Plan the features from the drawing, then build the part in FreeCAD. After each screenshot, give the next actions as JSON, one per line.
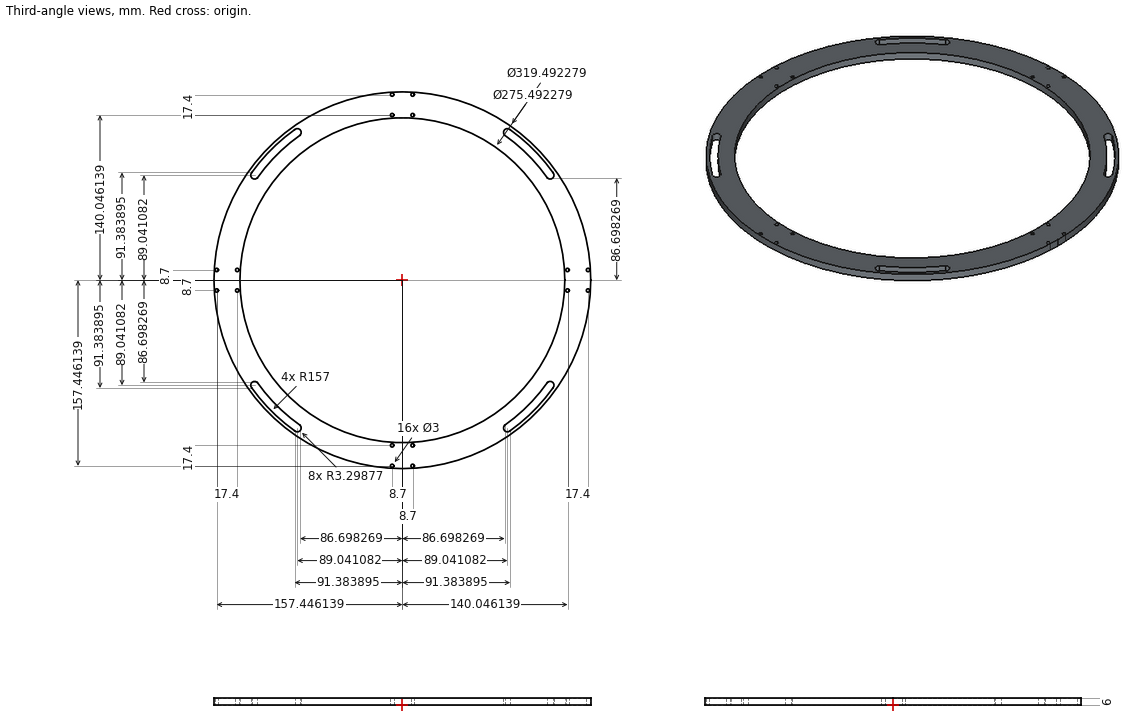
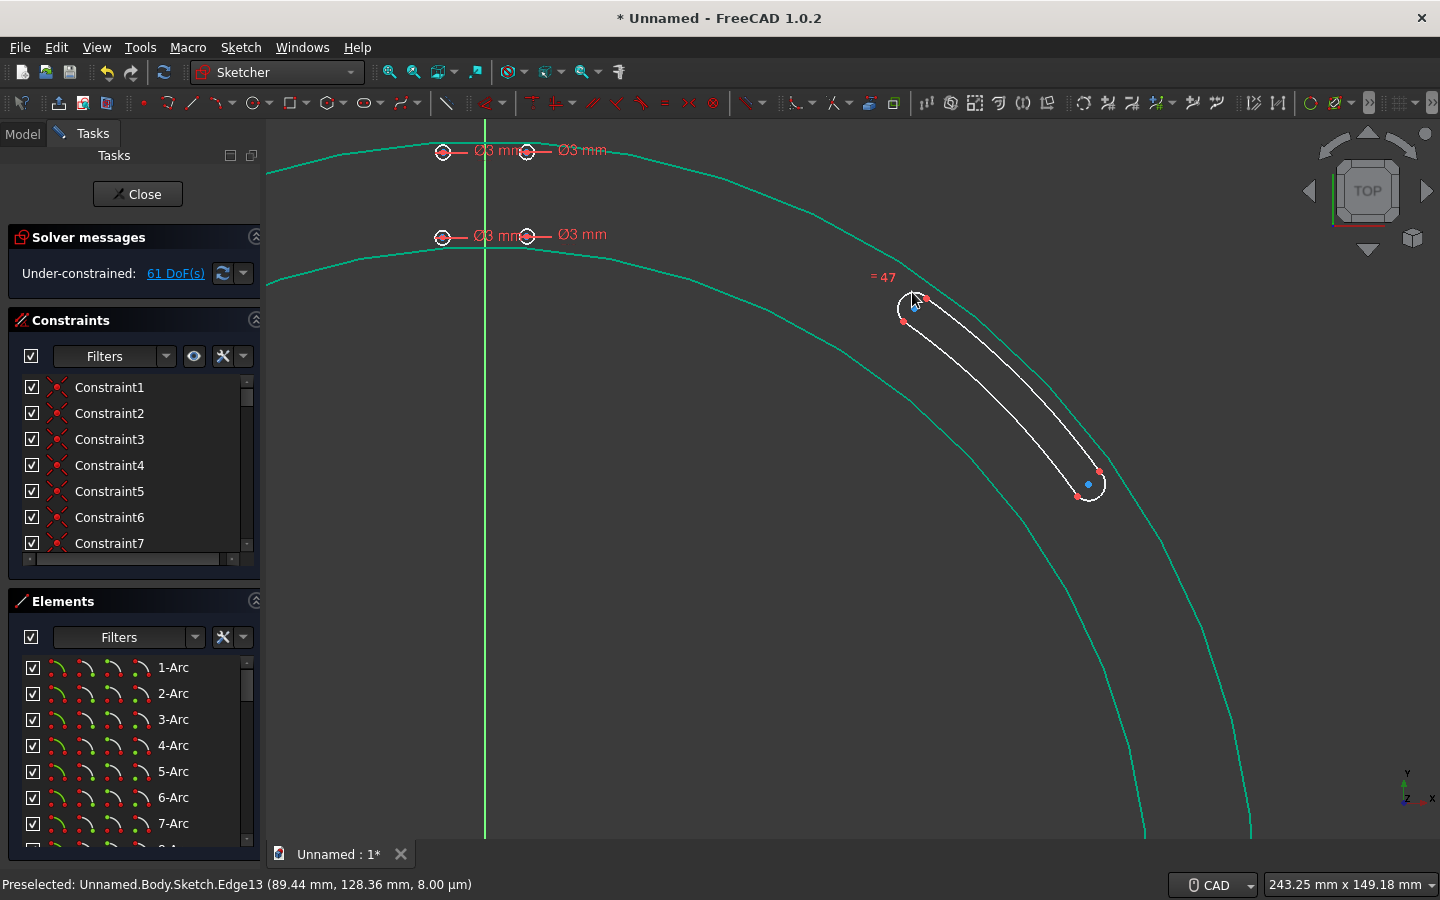
{"action": "scroll", "coordinate": [914, 292], "scroll_direction": "down", "scroll_amount": 6}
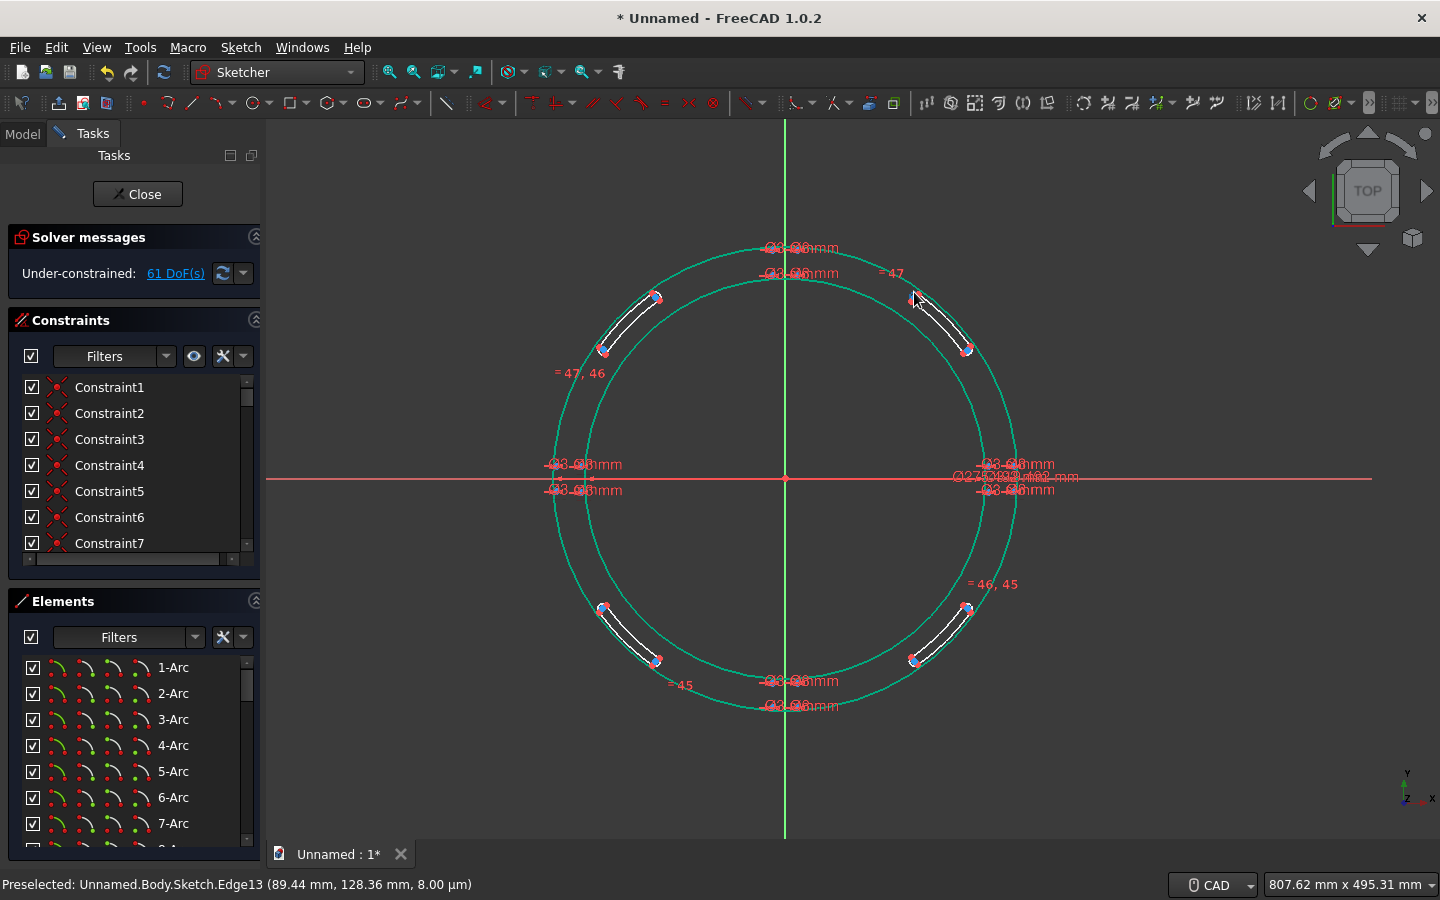
{"action": "scroll", "coordinate": [613, 630], "scroll_direction": "up", "scroll_amount": 7}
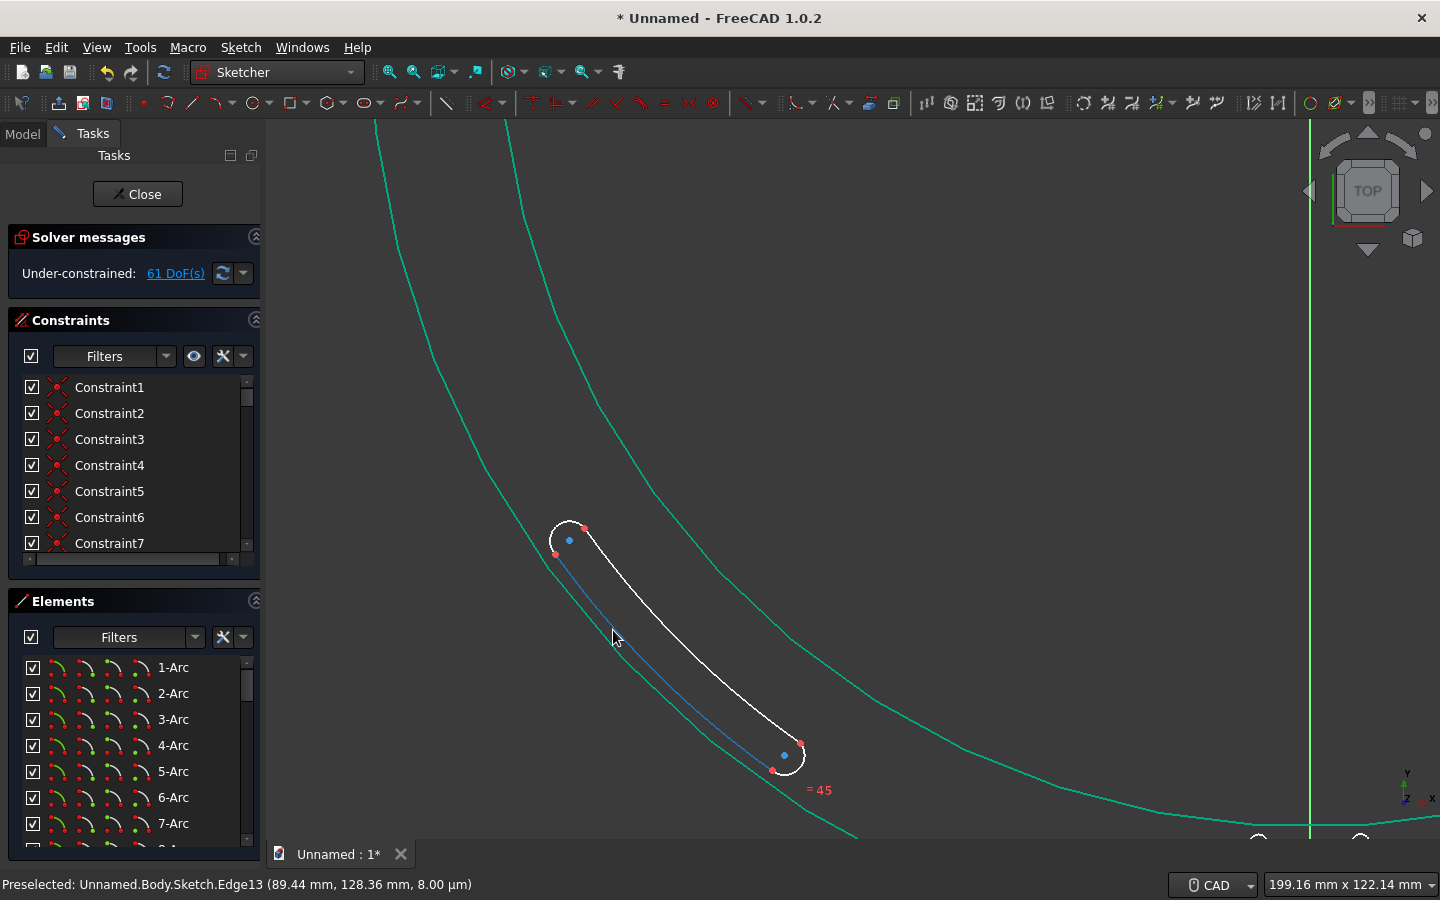
{"action": "left_click", "coordinate": [613, 627]}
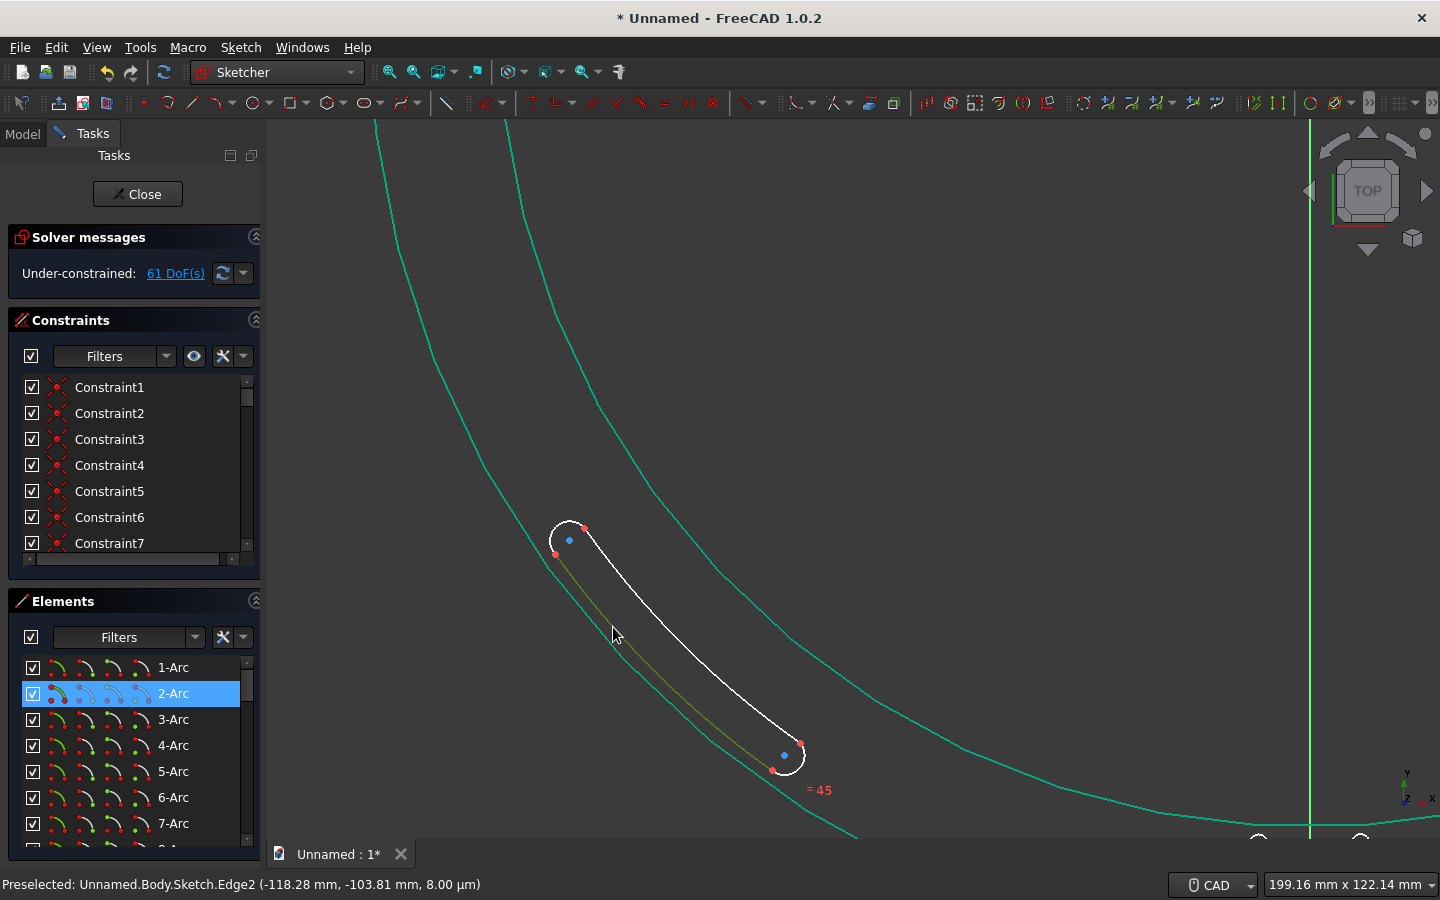
{"action": "scroll", "coordinate": [612, 631], "scroll_direction": "down", "scroll_amount": 7}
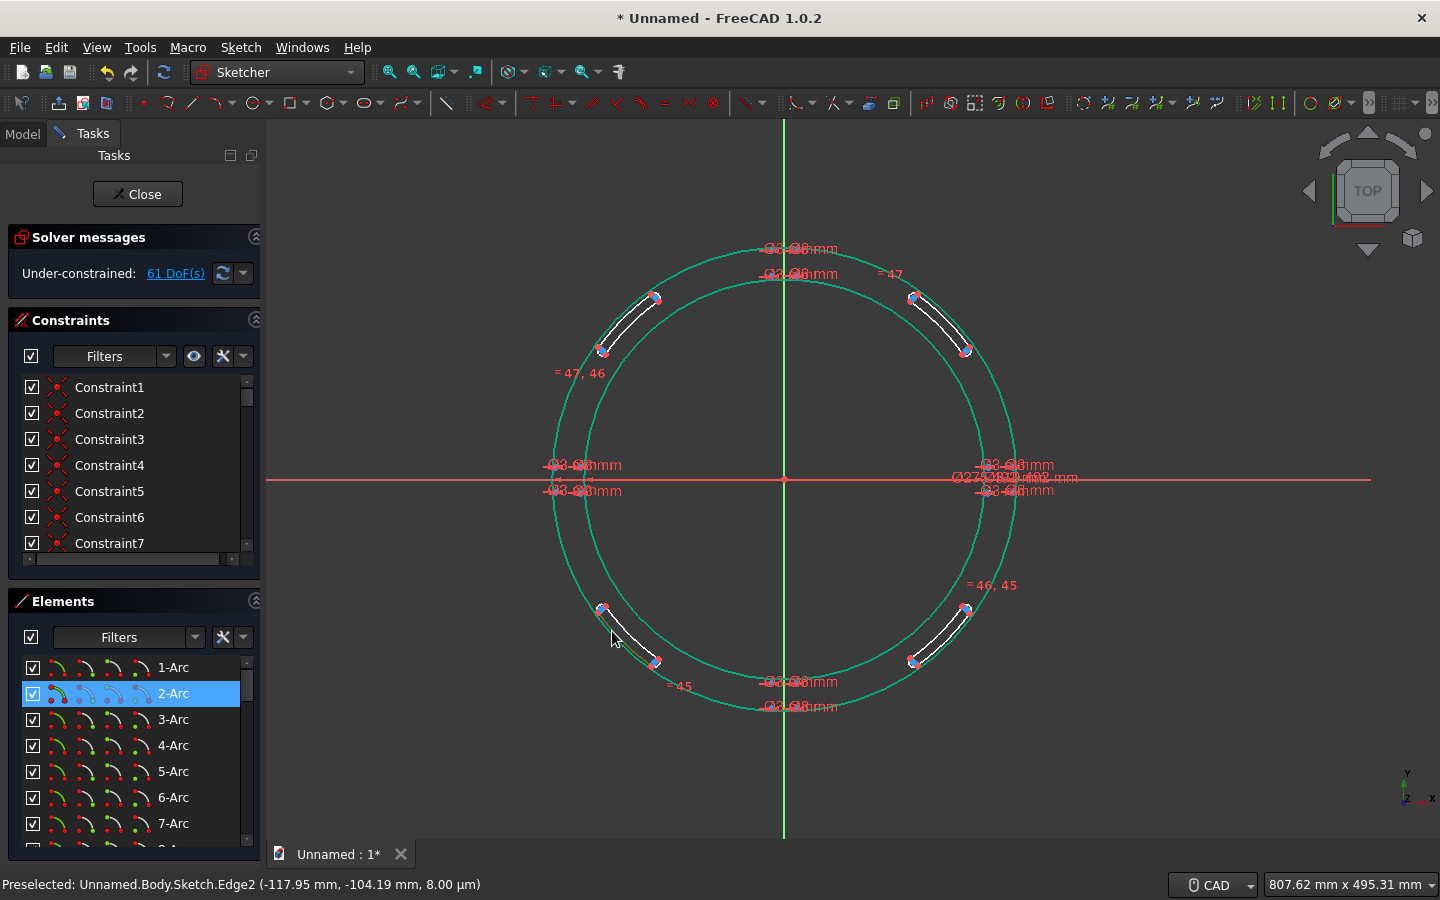
{"action": "scroll", "coordinate": [935, 652], "scroll_direction": "up", "scroll_amount": 7}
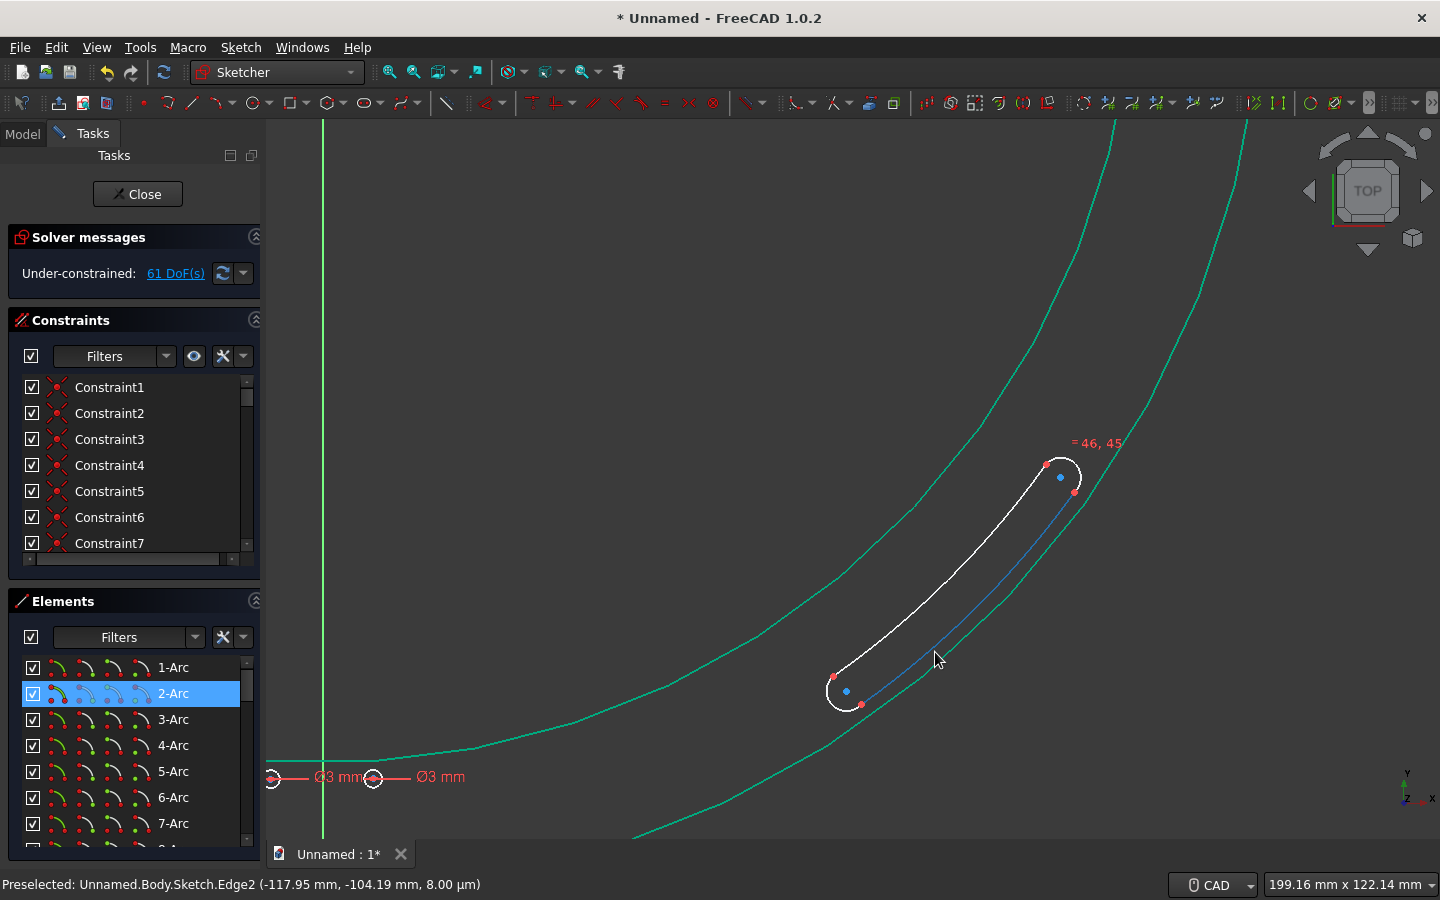
{"action": "left_click", "coordinate": [932, 649]}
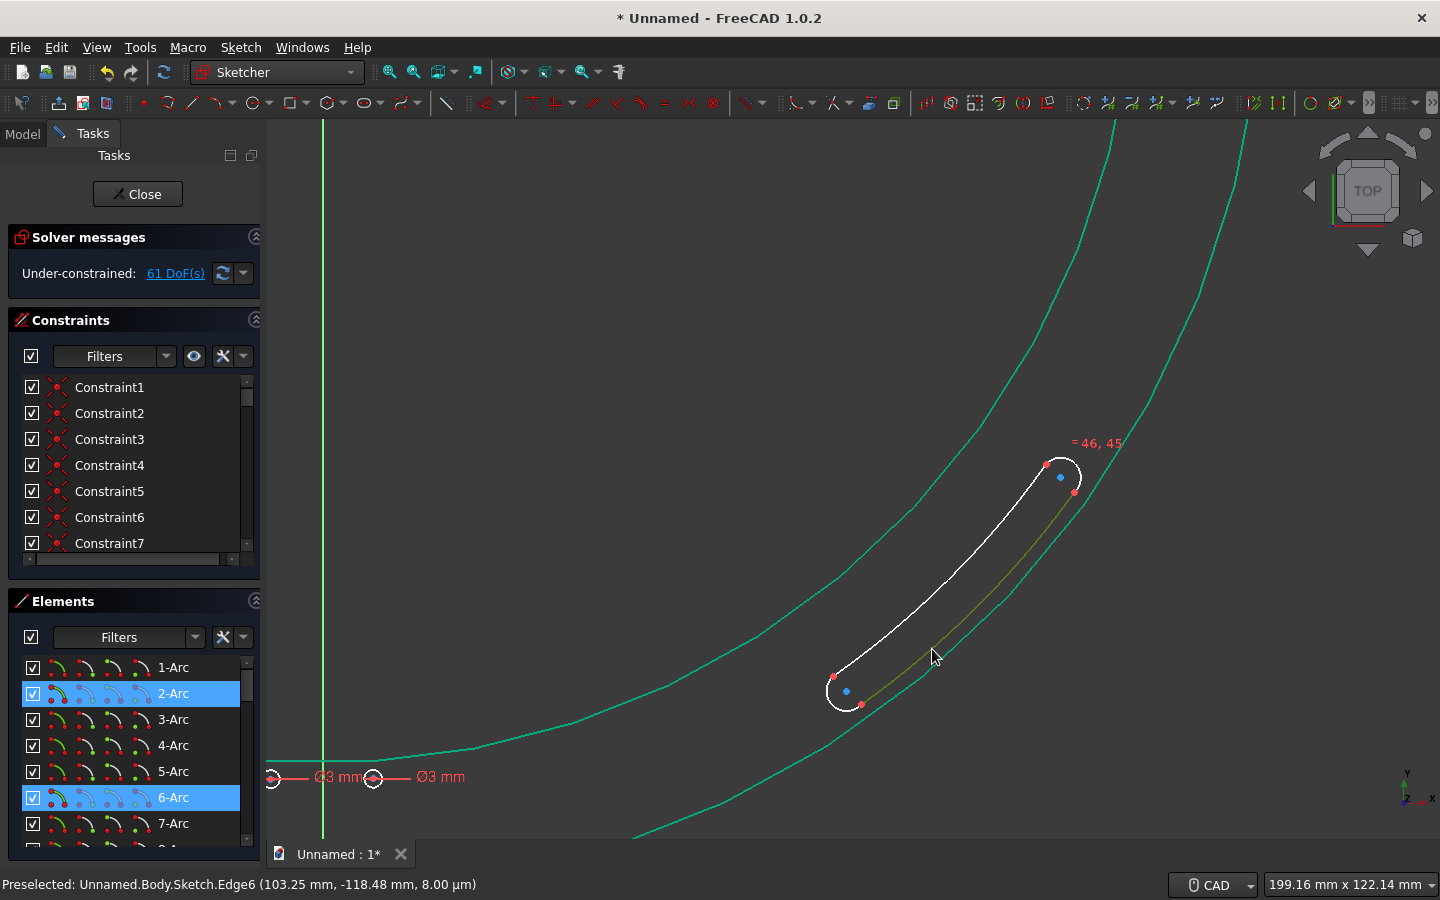
{"action": "scroll", "coordinate": [936, 652], "scroll_direction": "down", "scroll_amount": 7}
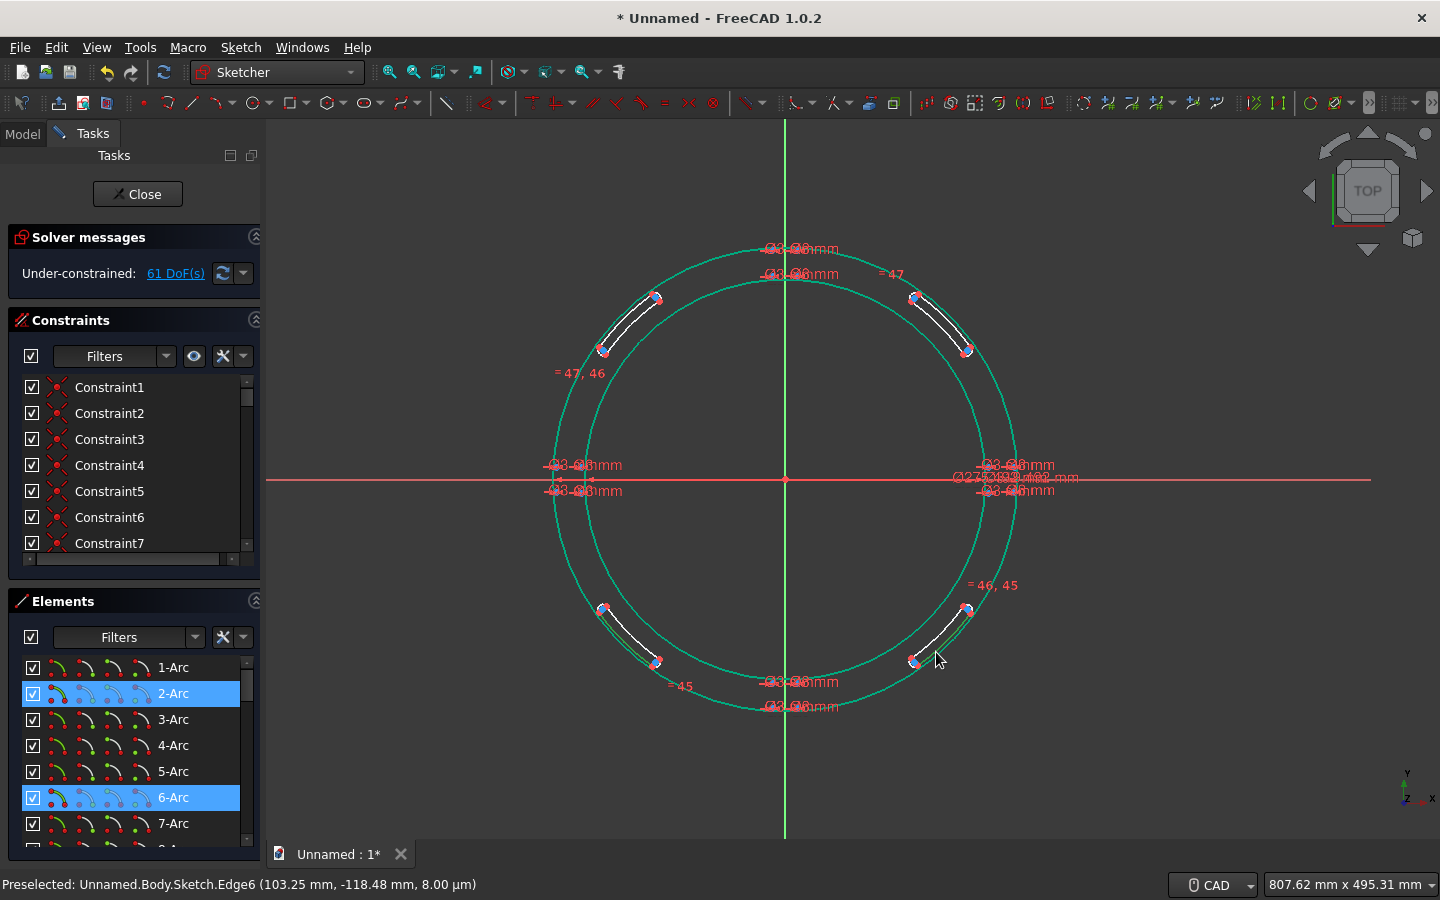
{"action": "scroll", "coordinate": [634, 309], "scroll_direction": "up", "scroll_amount": 6}